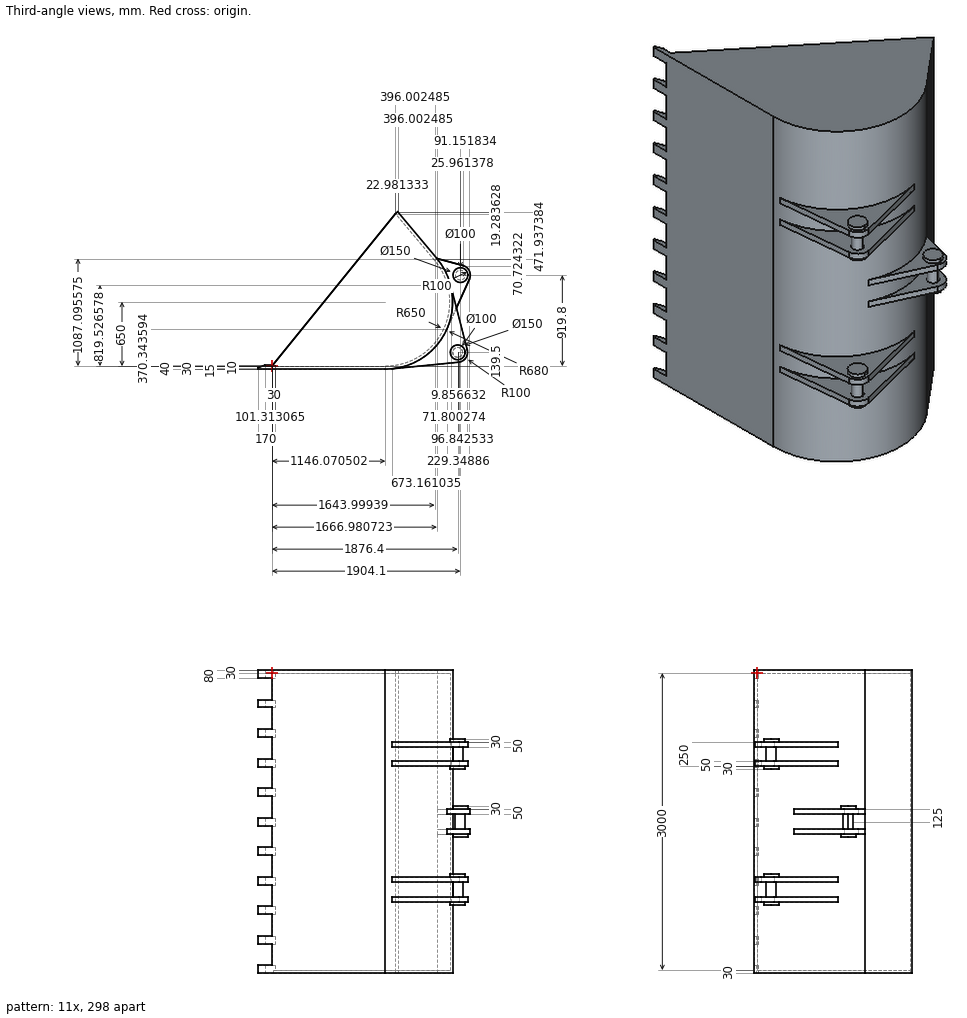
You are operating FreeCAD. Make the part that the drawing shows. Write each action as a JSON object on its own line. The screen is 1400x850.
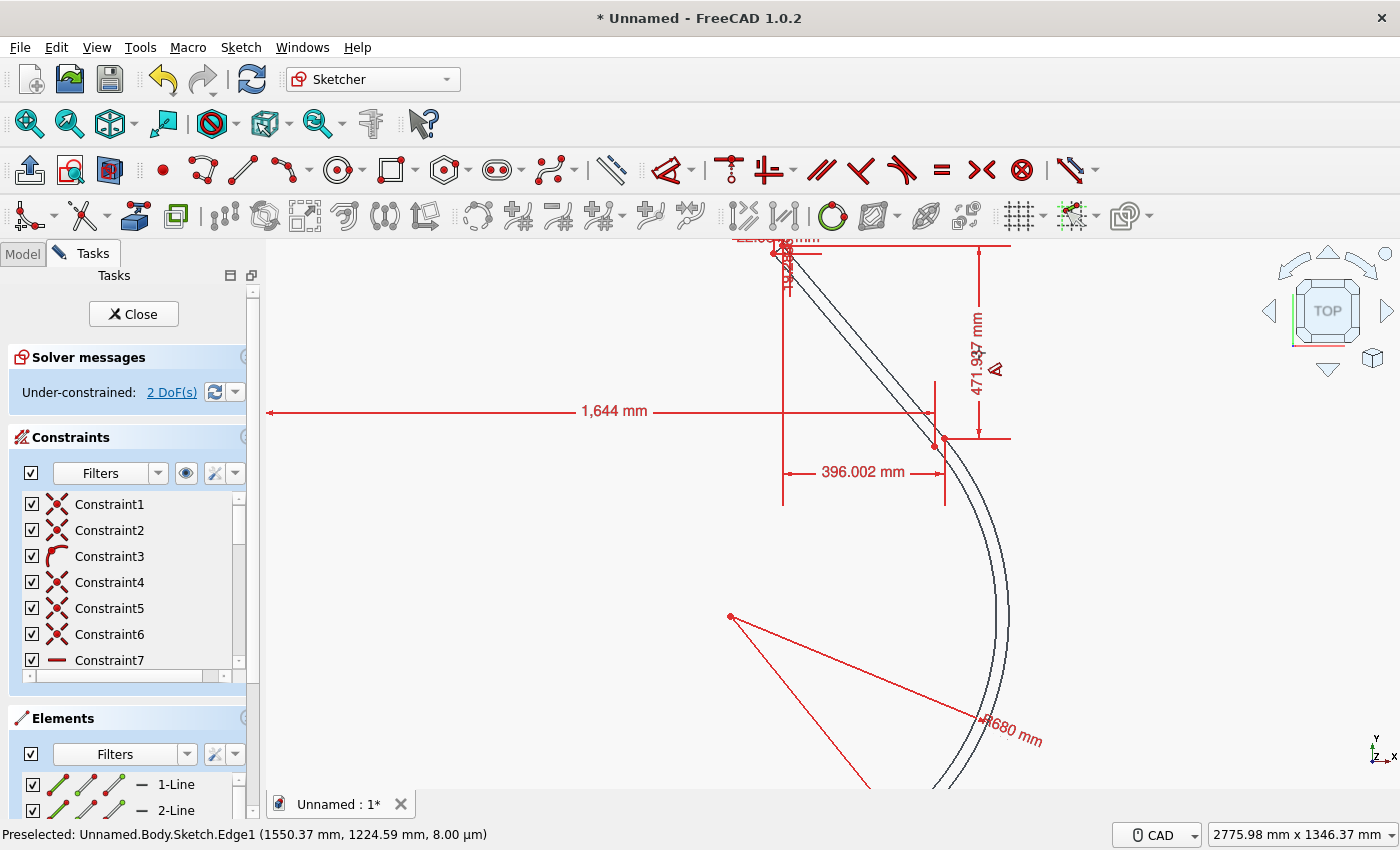
{"action": "left_click", "coordinate": [822, 312]}
{"action": "left_click", "coordinate": [854, 504]}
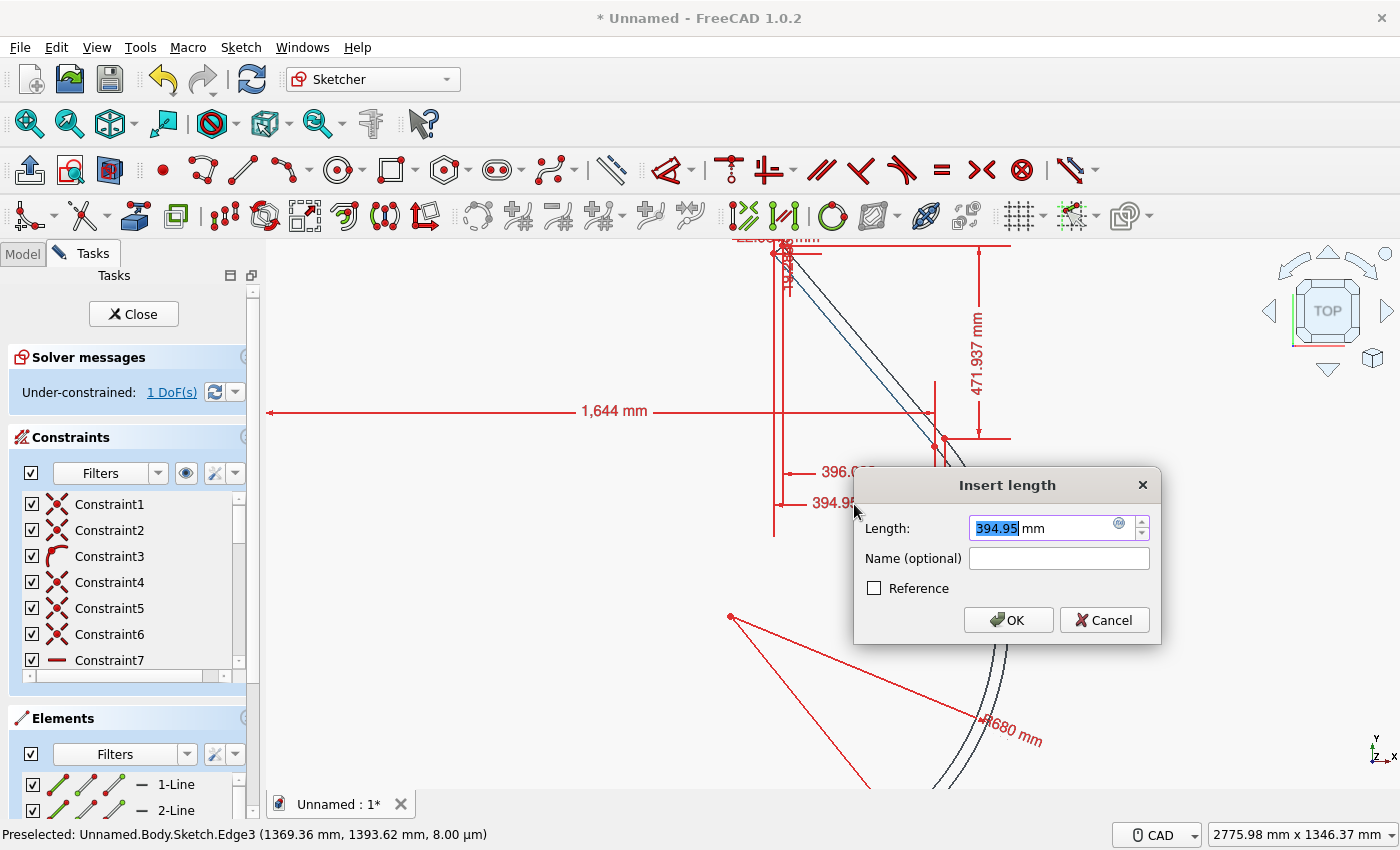
{"action": "type", "text": "396.002485"}
{"action": "key", "text": "Return"}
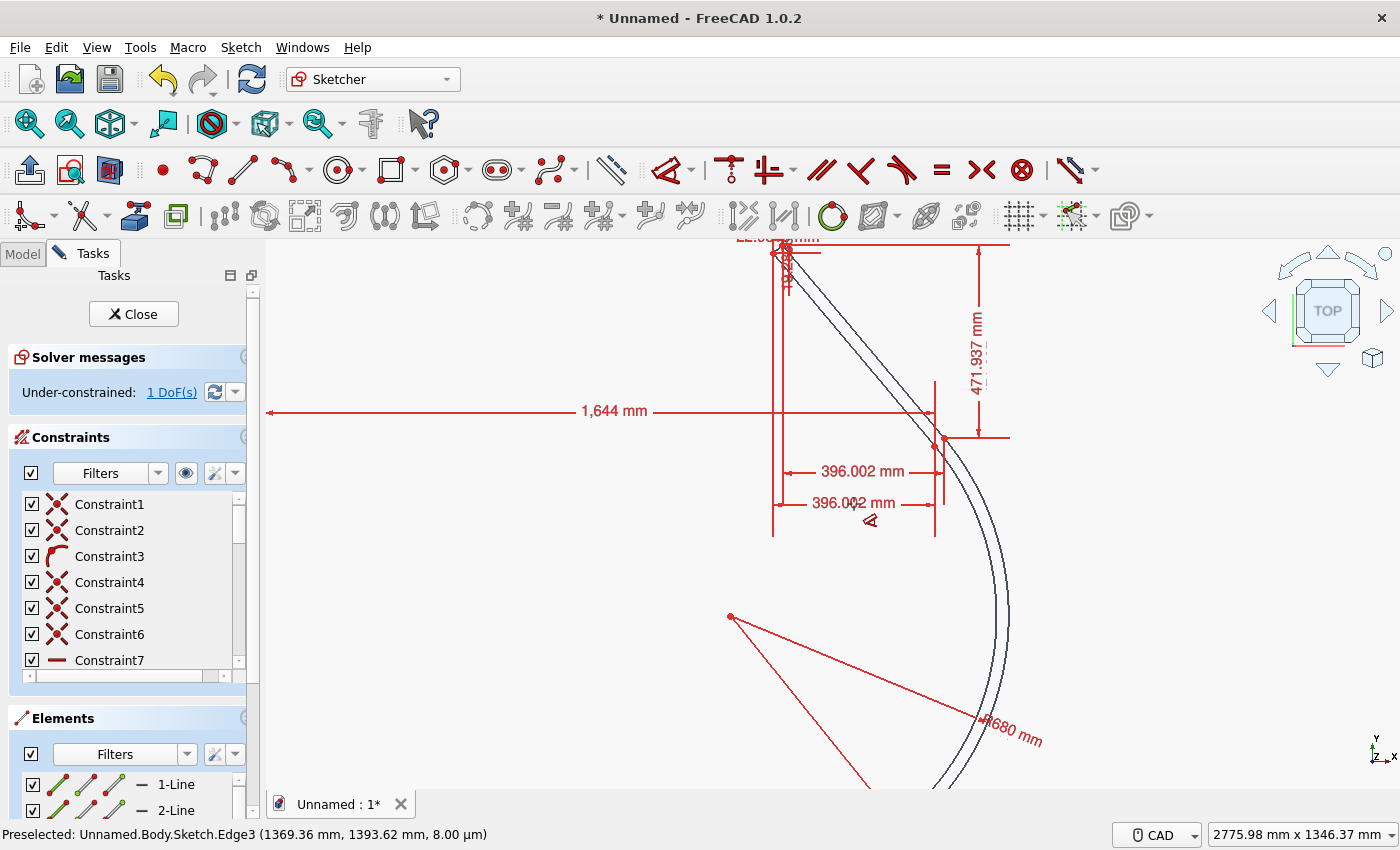
{"action": "left_click", "coordinate": [944, 438]}
{"action": "left_click", "coordinate": [978, 600]}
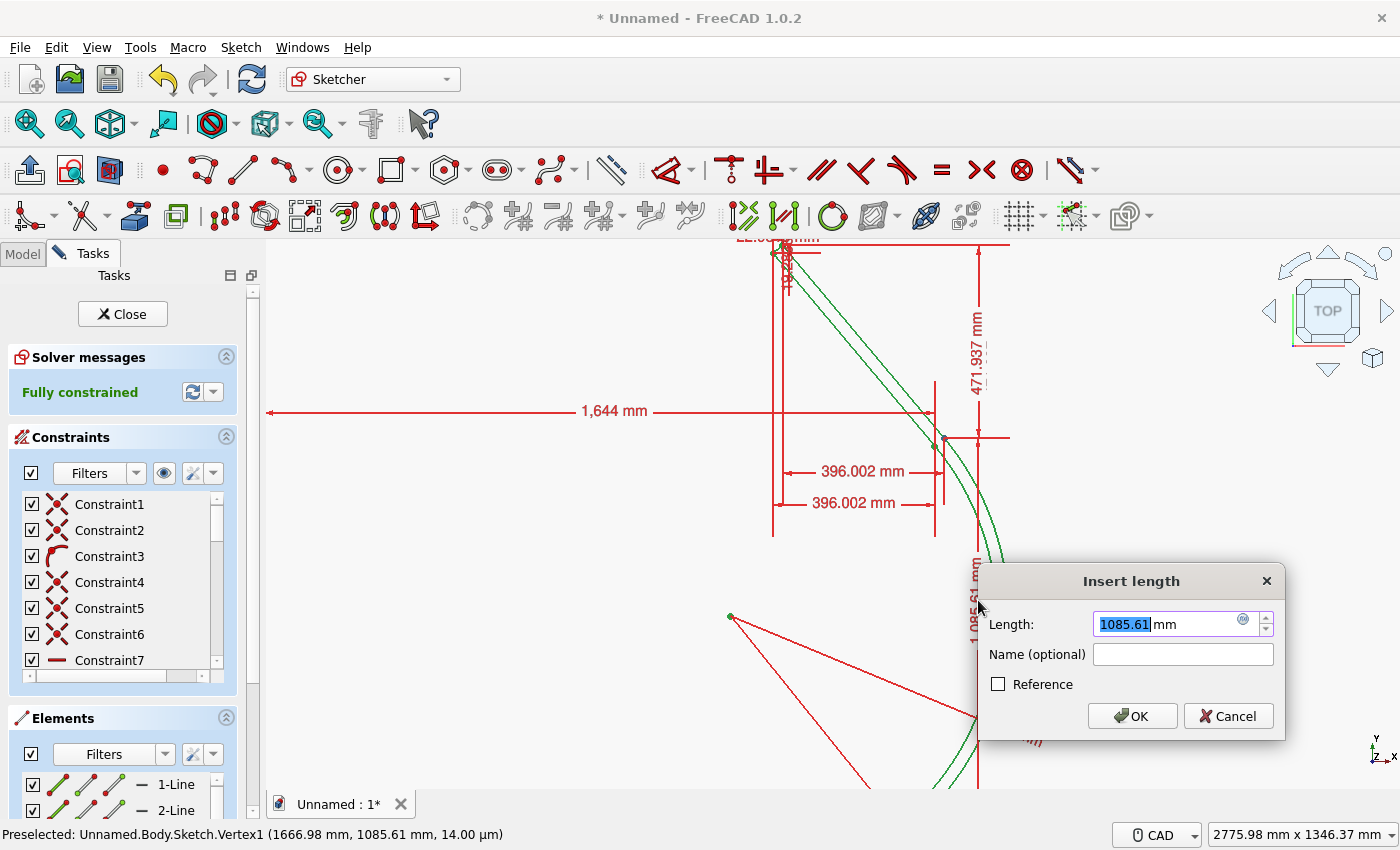
{"action": "type", "text": "1087.095575"}
{"action": "key", "text": "Return"}
{"action": "key", "text": "Escape"}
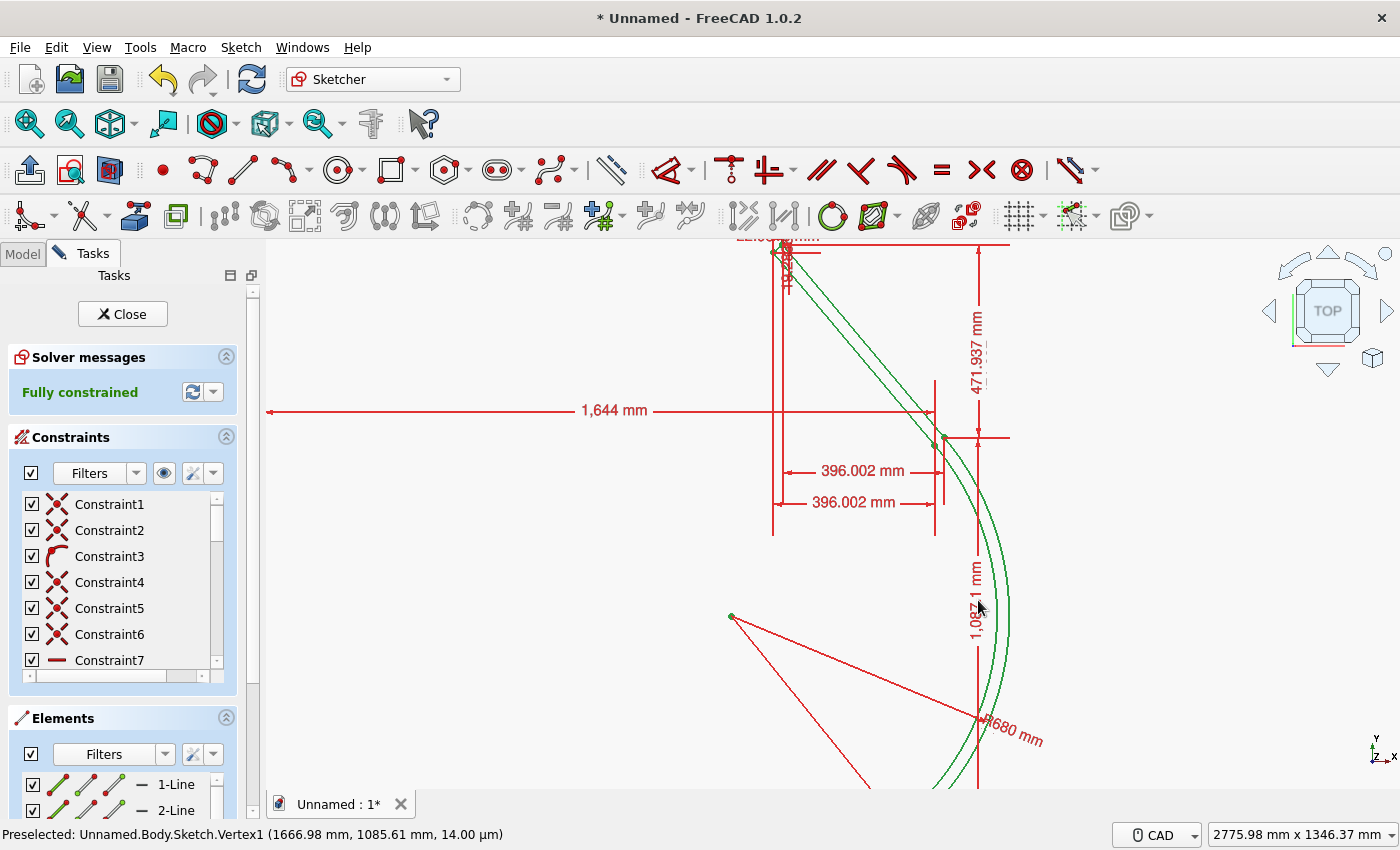
{"action": "left_click", "coordinate": [123, 314]}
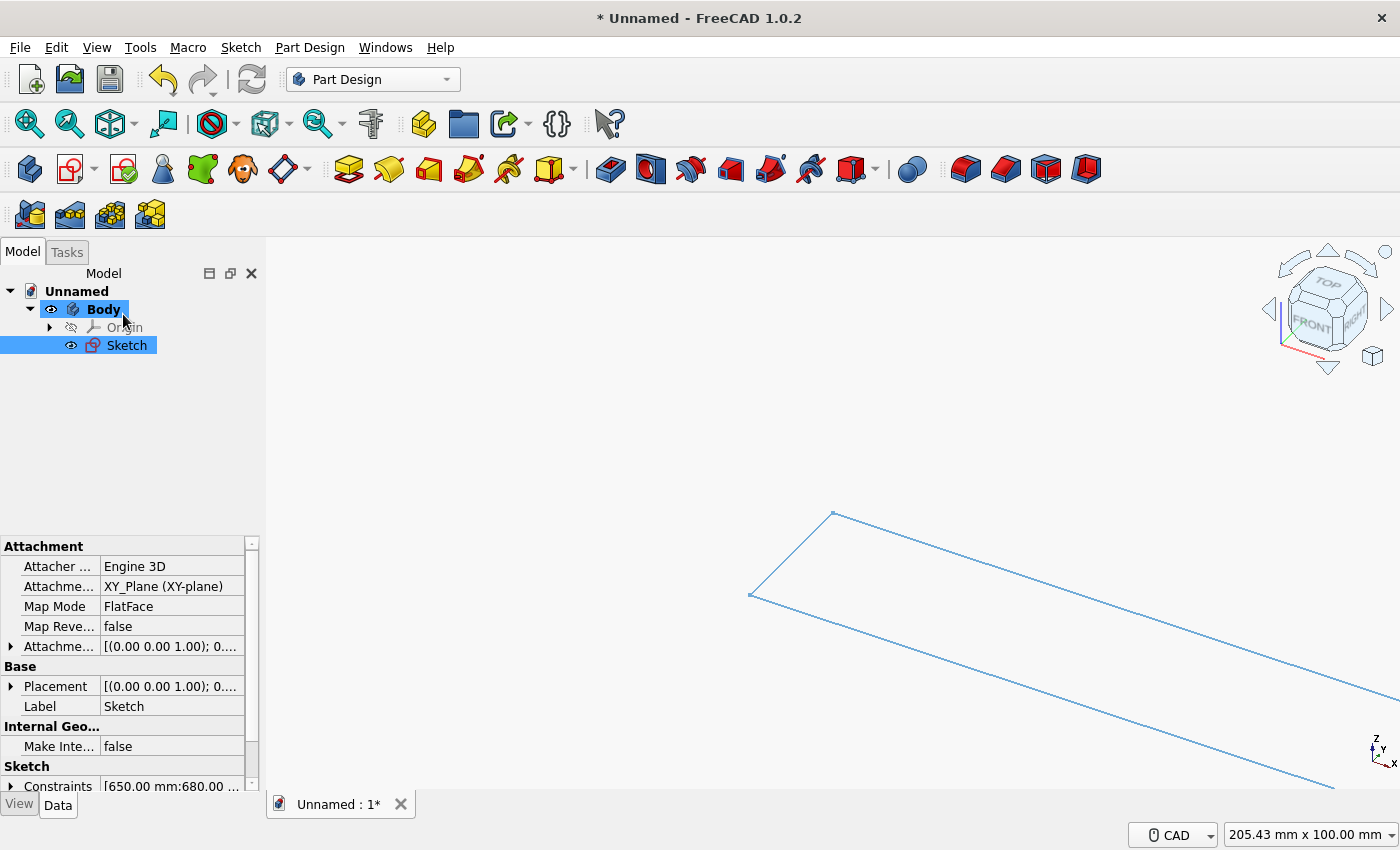
{"action": "left_click", "coordinate": [350, 170]}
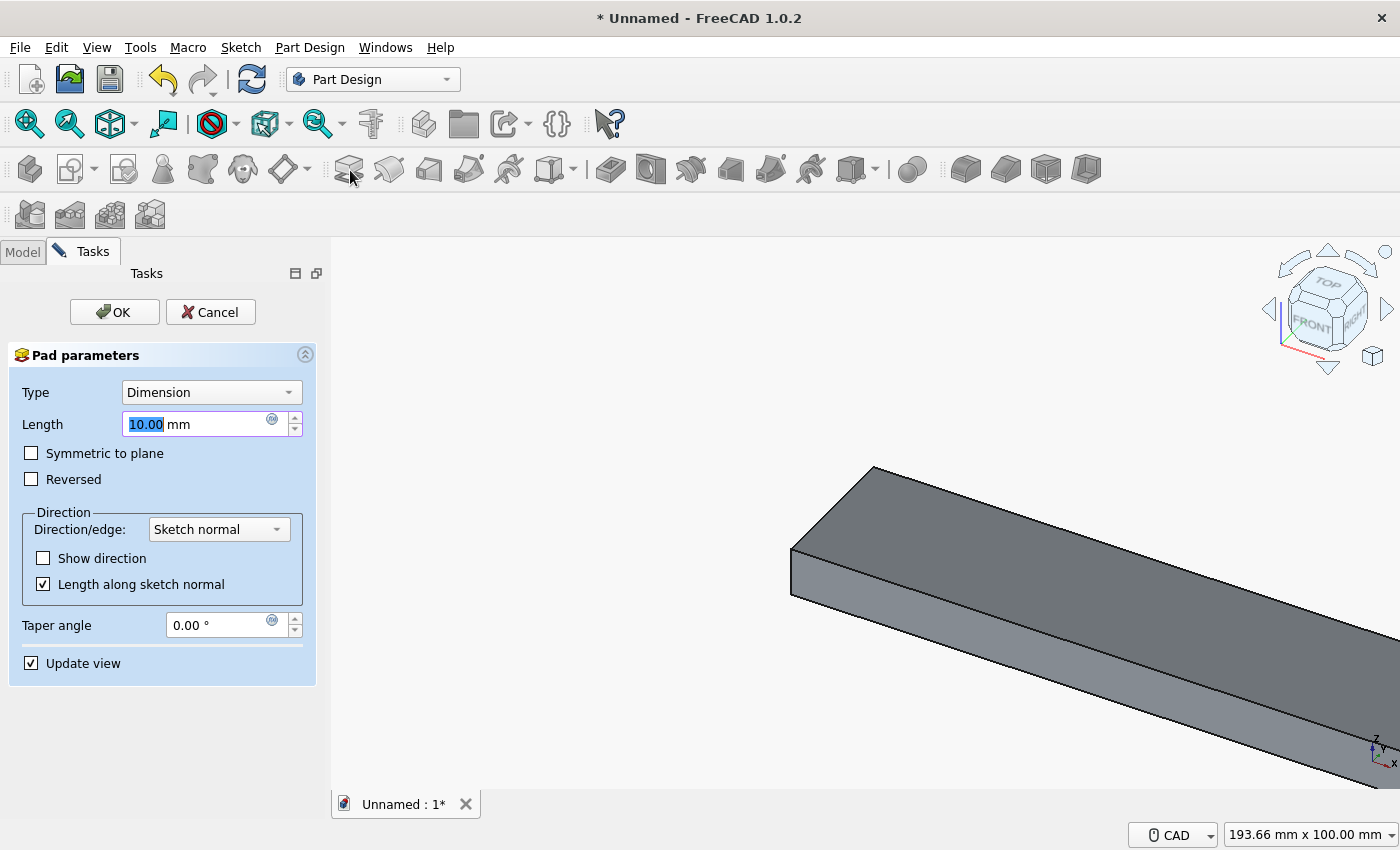
{"action": "type", "text": "3000"}
{"action": "key", "text": "Tab"}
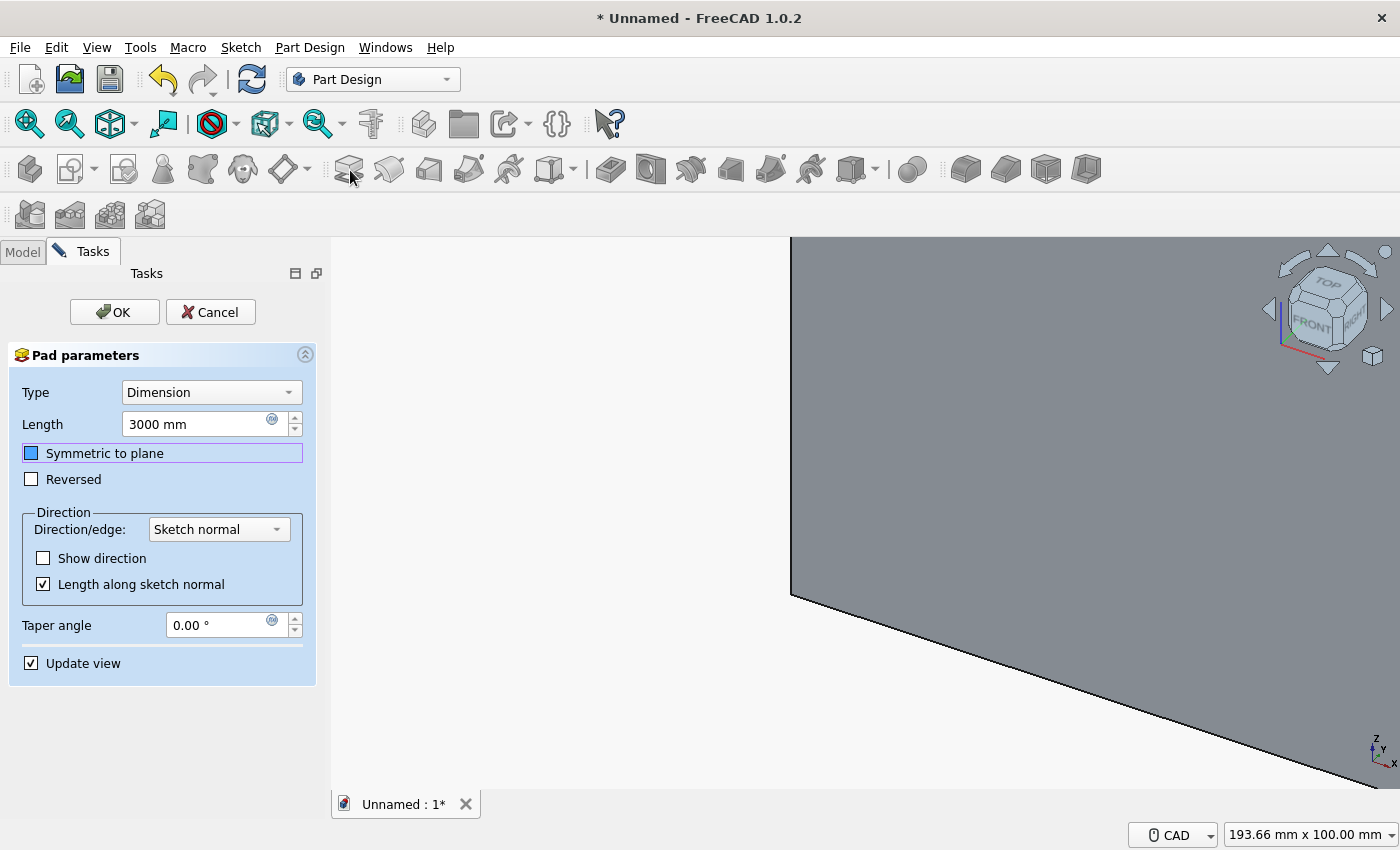
{"action": "left_click", "coordinate": [30, 479]}